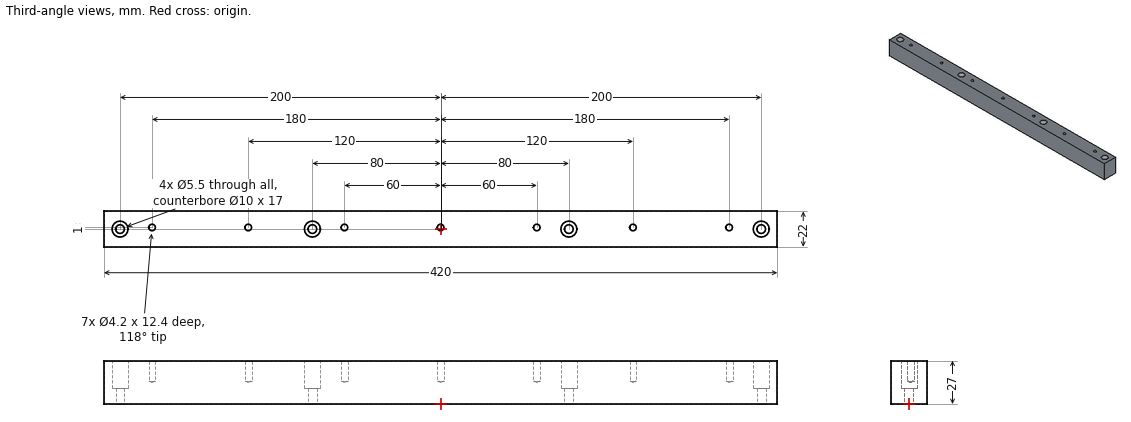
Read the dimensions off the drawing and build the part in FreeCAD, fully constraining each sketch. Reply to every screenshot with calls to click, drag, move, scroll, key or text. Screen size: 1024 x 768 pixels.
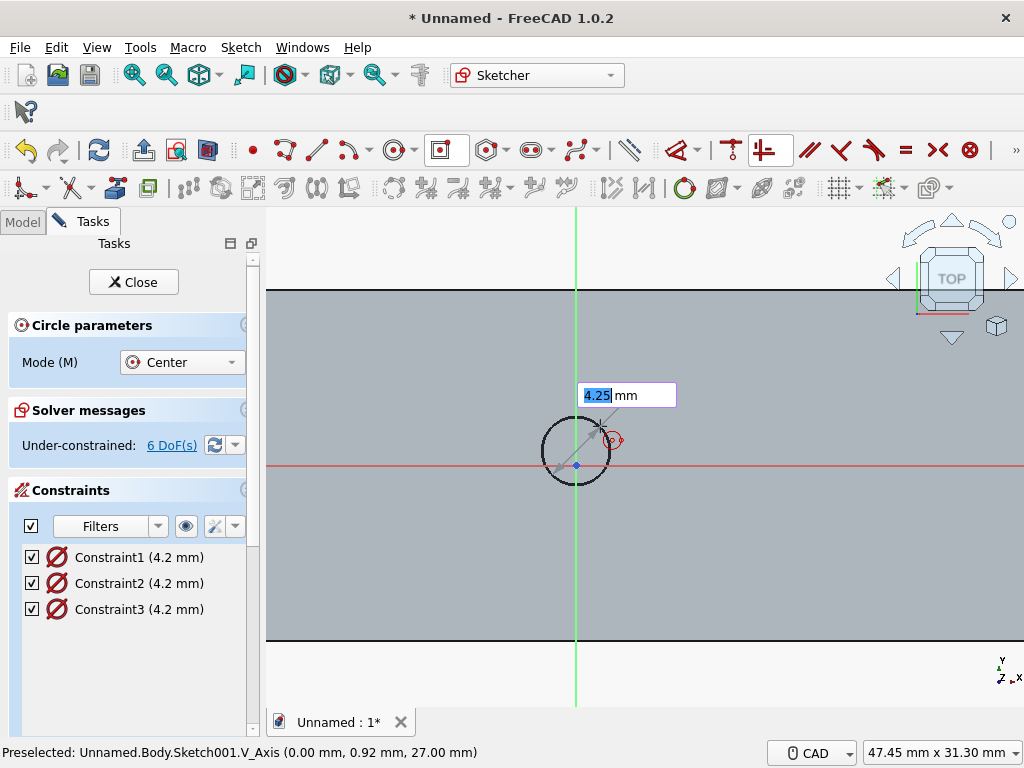
text(4.2)
key(Return)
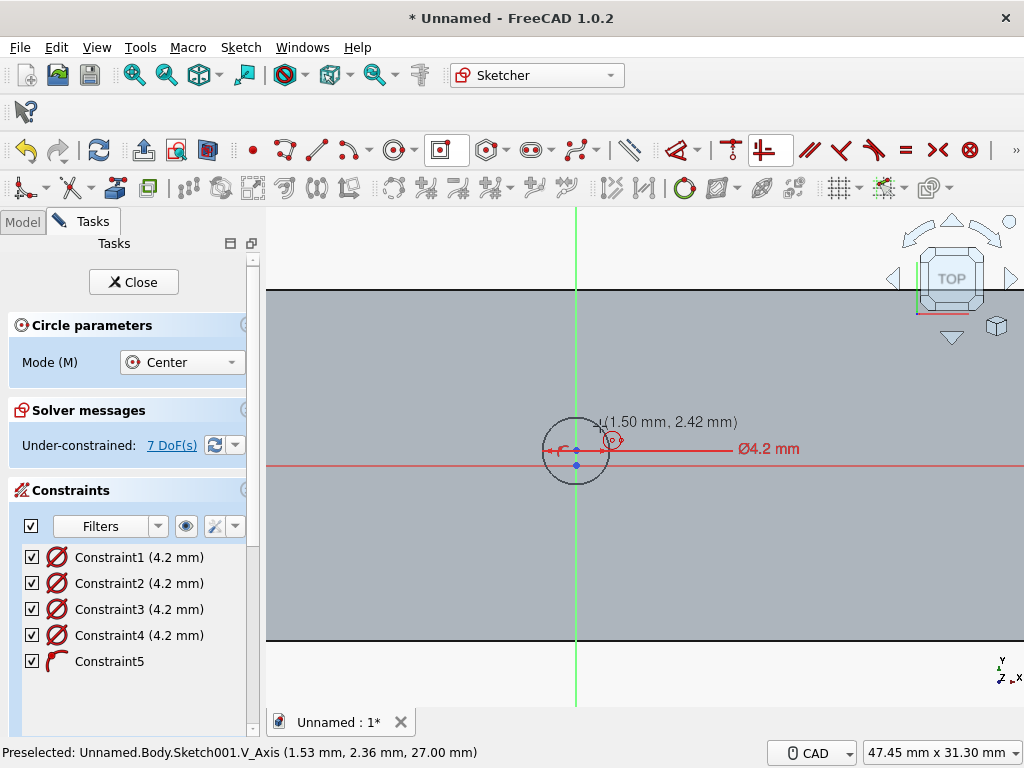
scroll(577, 458, down, 13)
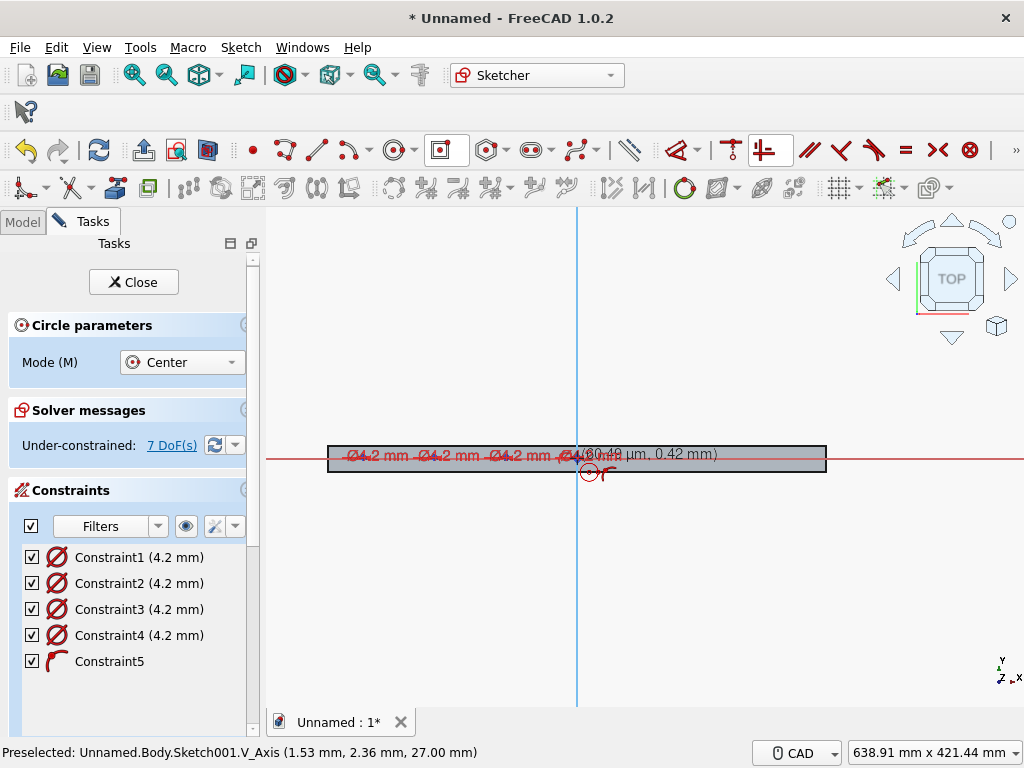
scroll(648, 458, up, 13)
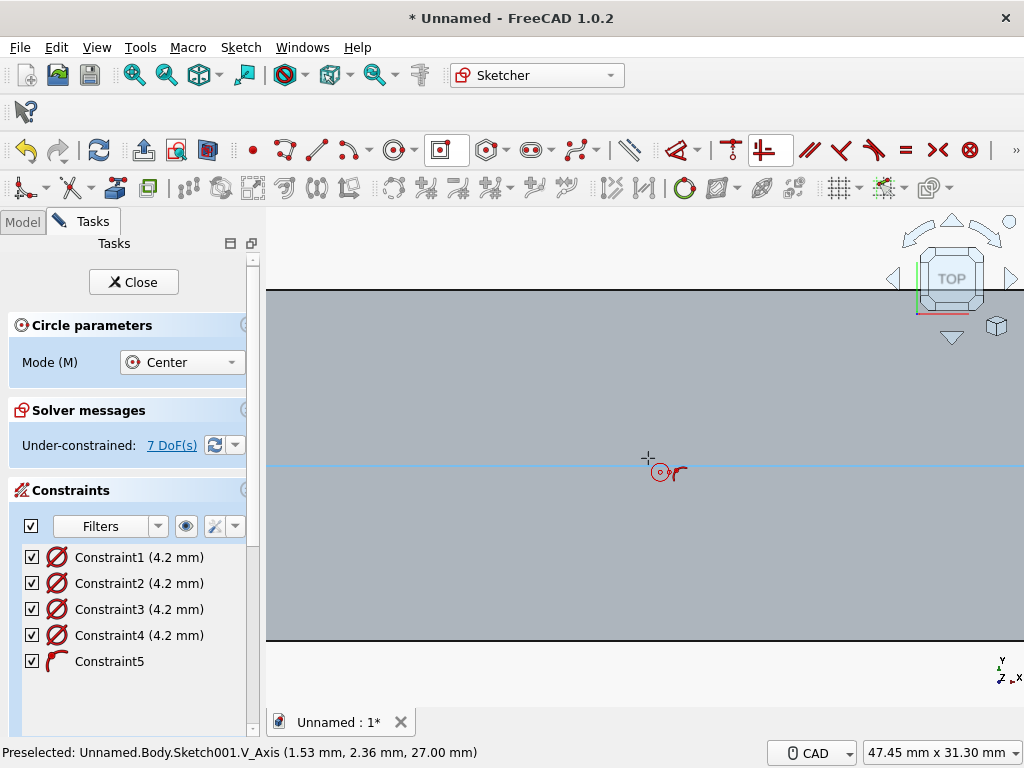
click(648, 450)
move(672, 426)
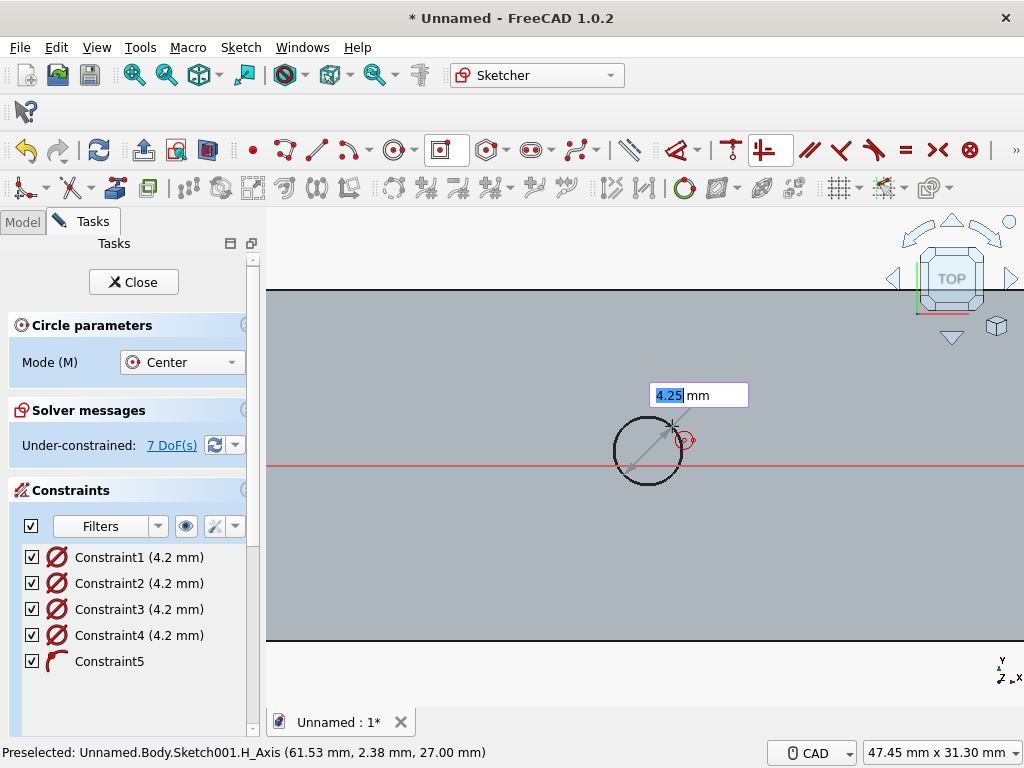
text(4.2)
key(Return)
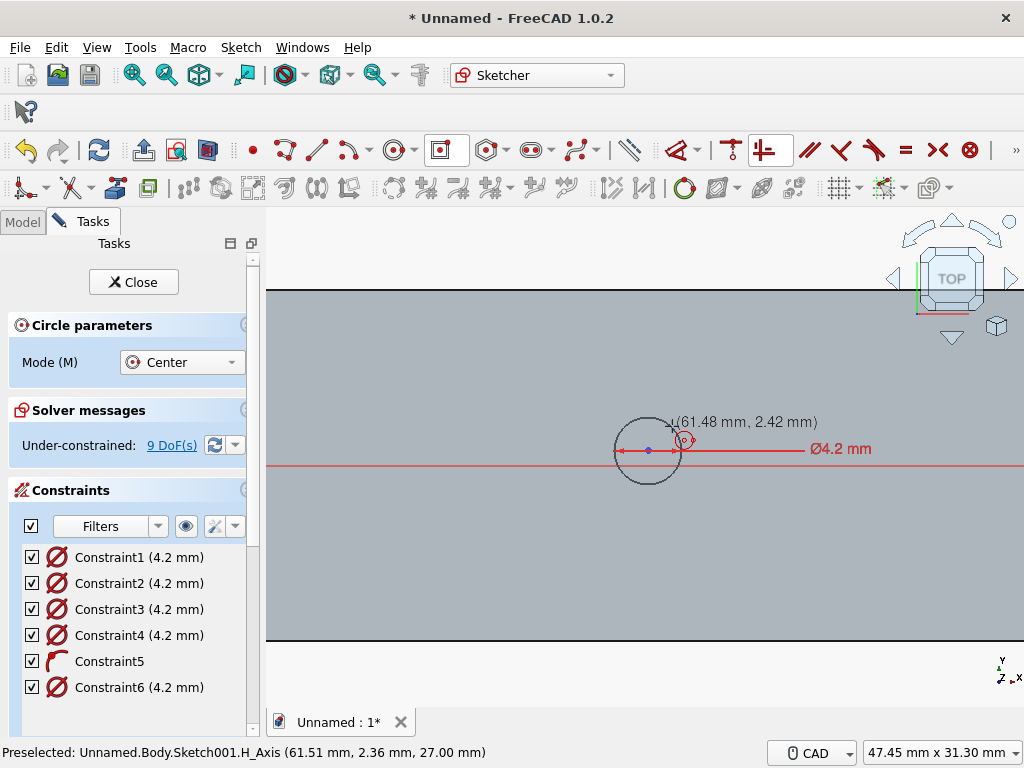
scroll(648, 458, down, 13)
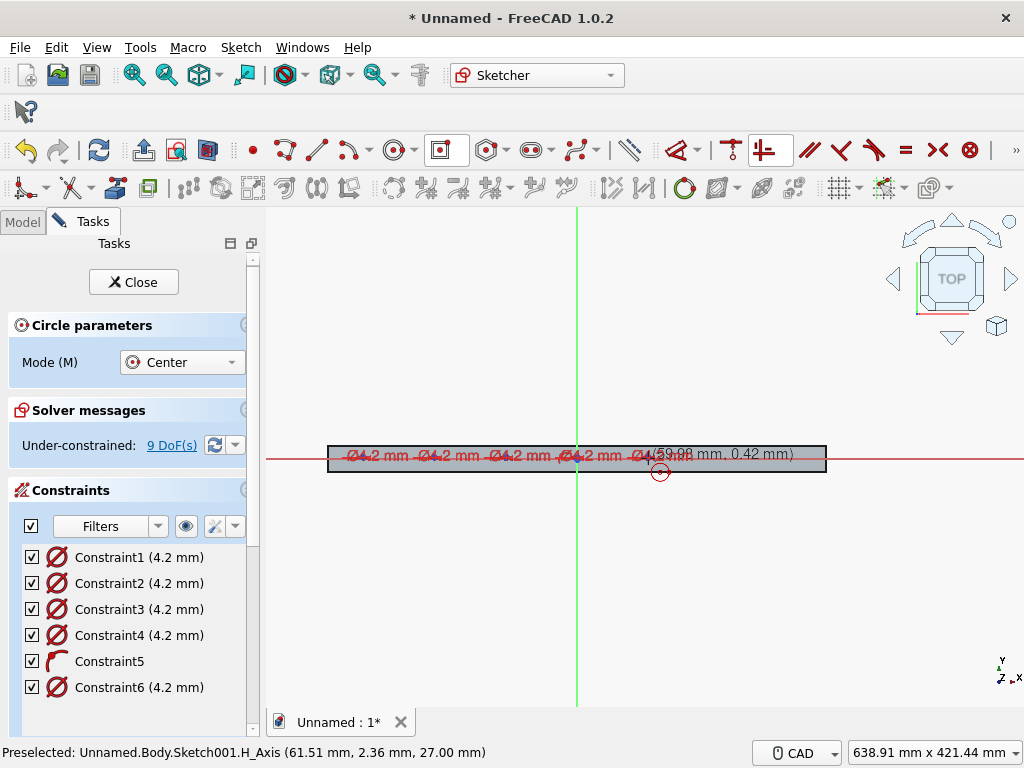
scroll(720, 458, up, 13)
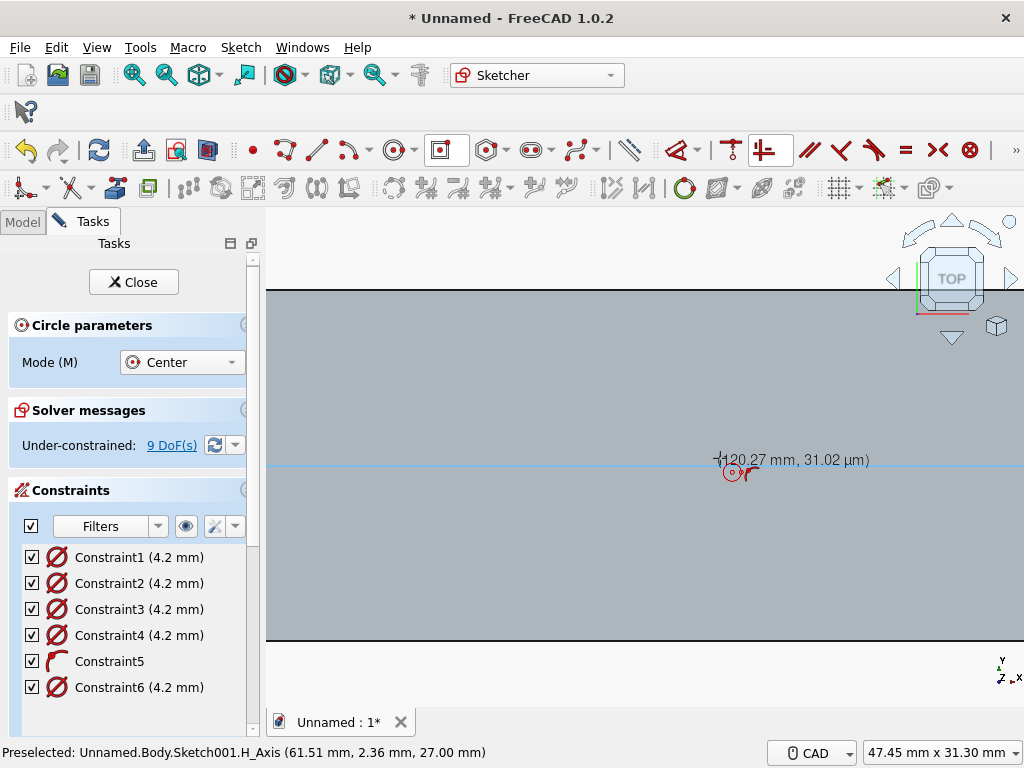
click(708, 450)
move(732, 426)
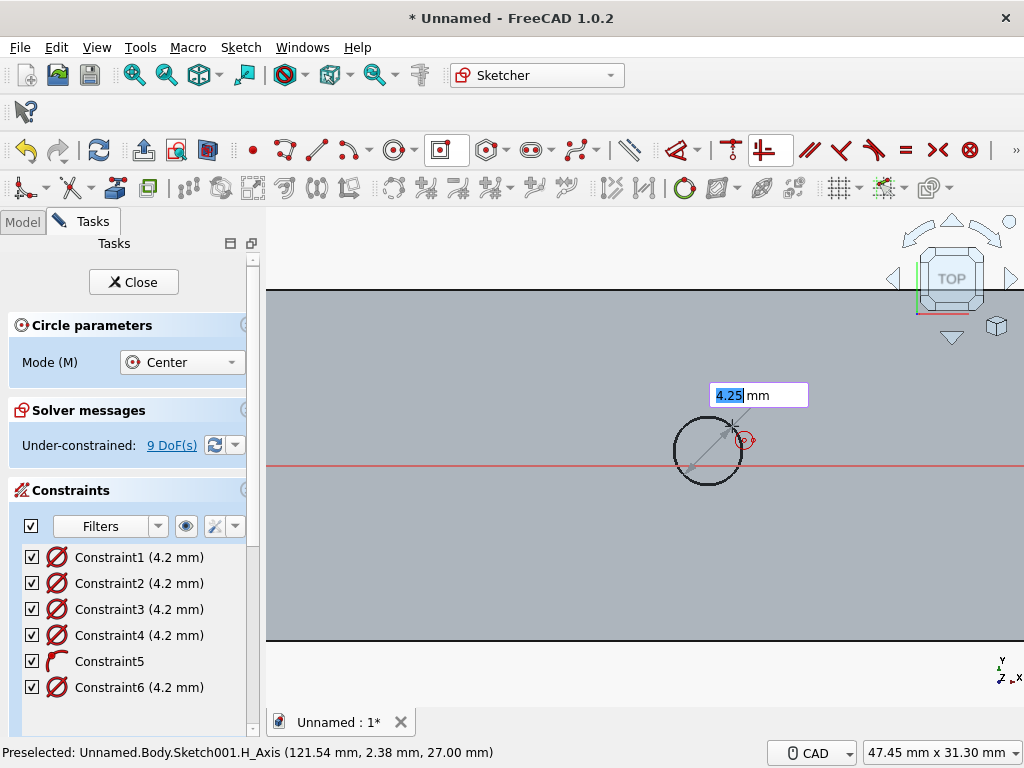
text(4.2)
key(Return)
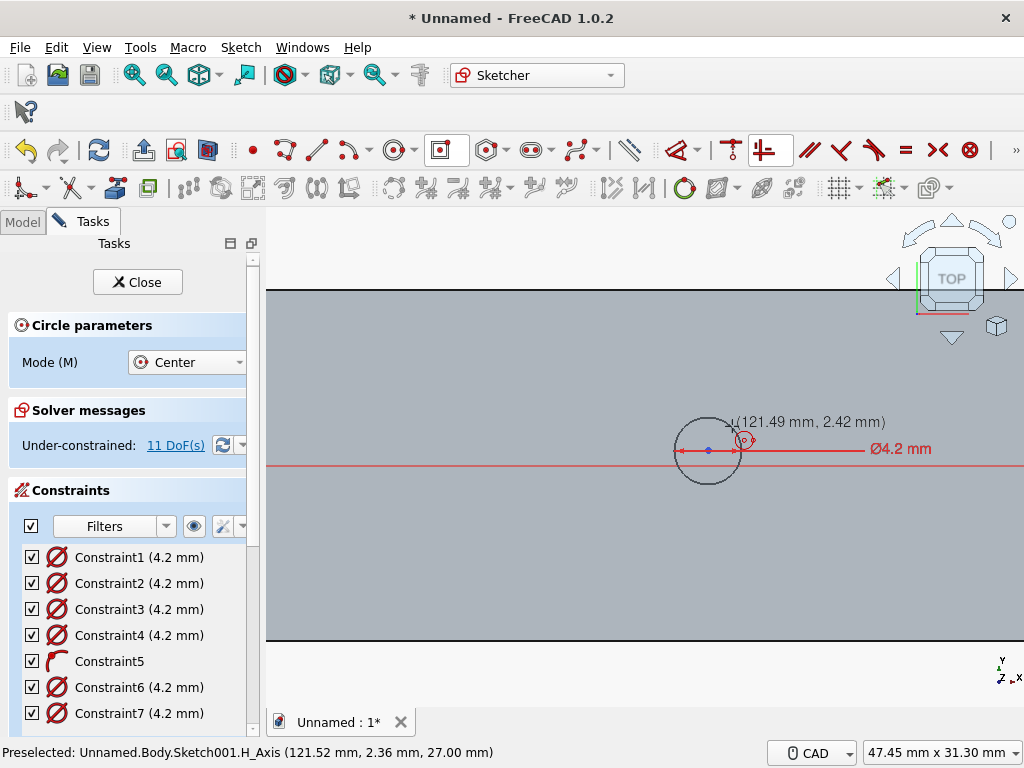
scroll(720, 458, down, 13)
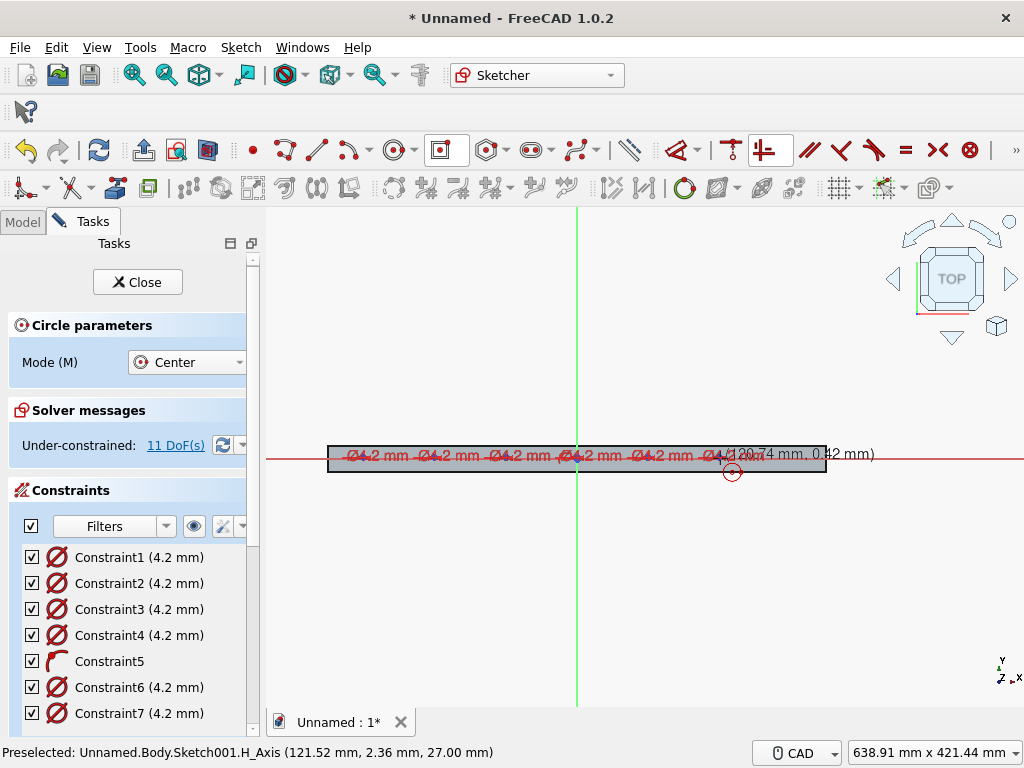
scroll(791, 458, up, 13)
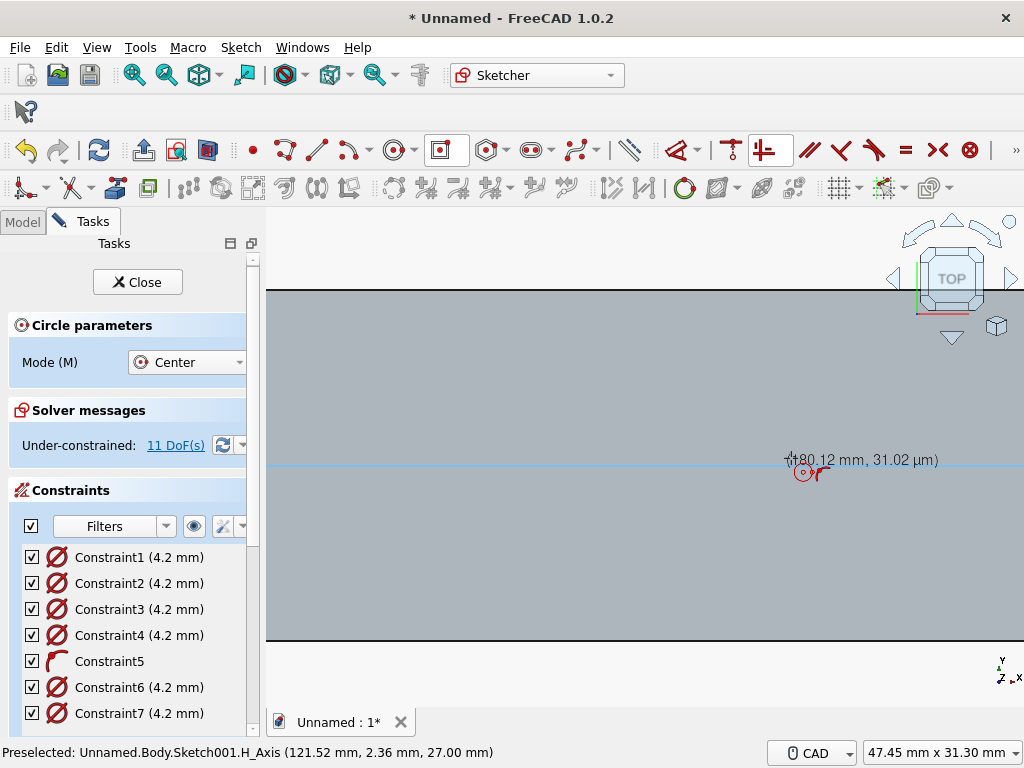
click(780, 450)
move(804, 426)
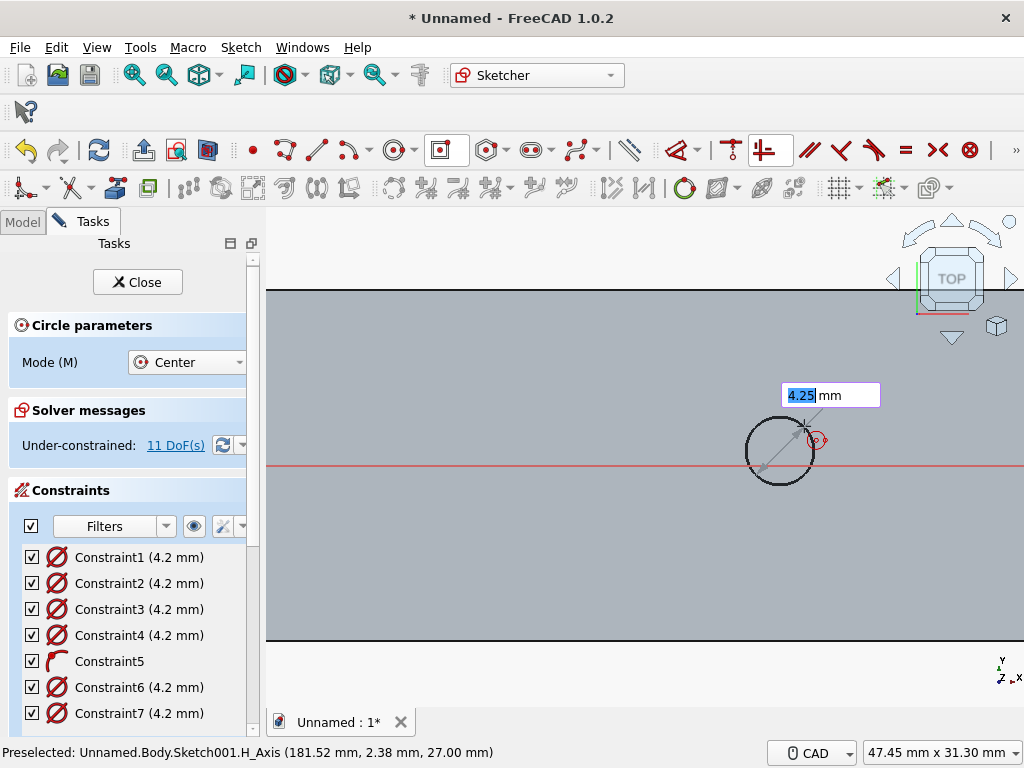
text(4.2)
key(Return)
key(Escape)